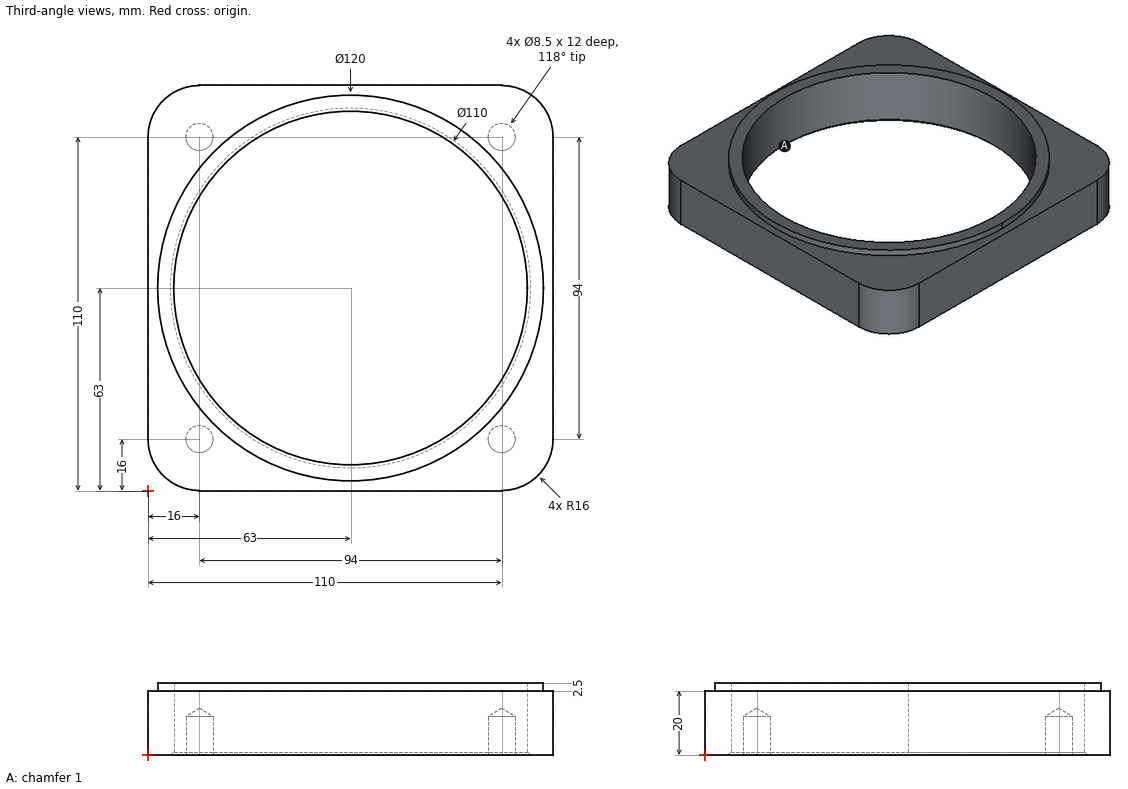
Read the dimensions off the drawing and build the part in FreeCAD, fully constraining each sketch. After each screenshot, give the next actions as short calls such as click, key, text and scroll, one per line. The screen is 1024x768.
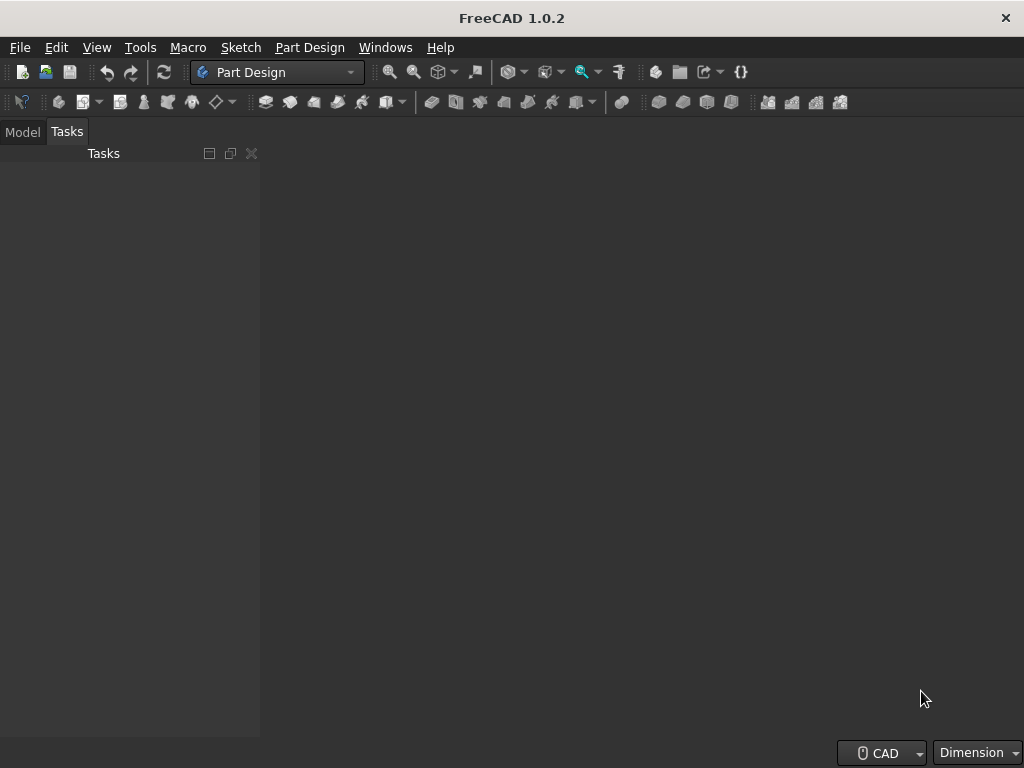
click(22, 72)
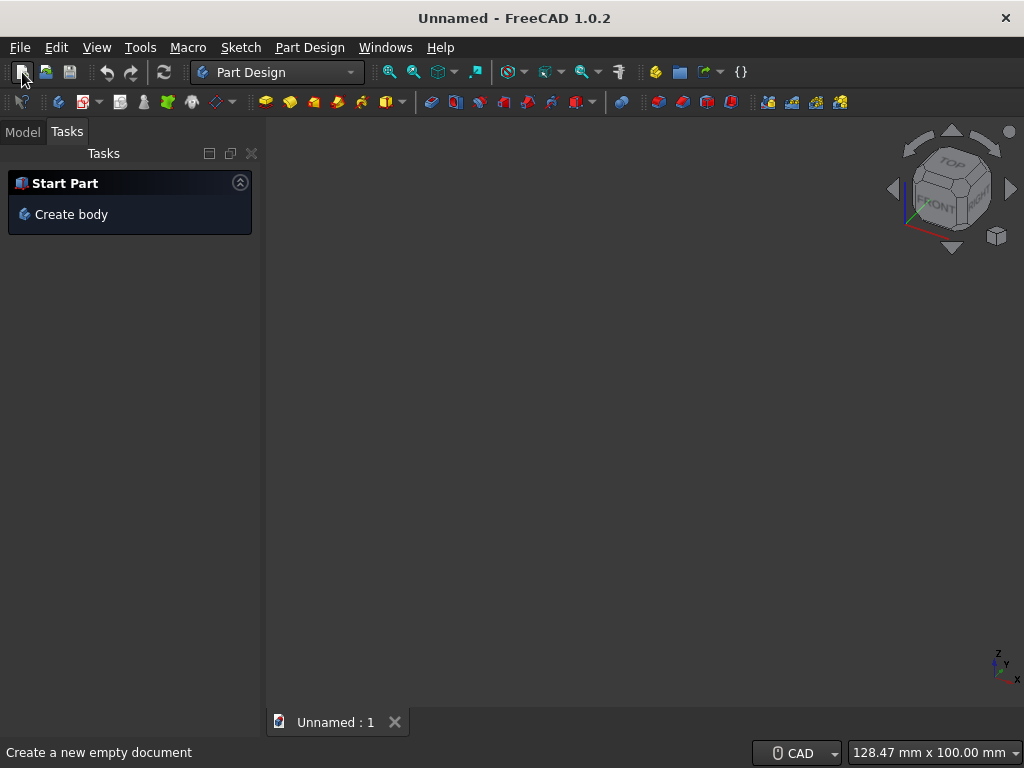
click(84, 102)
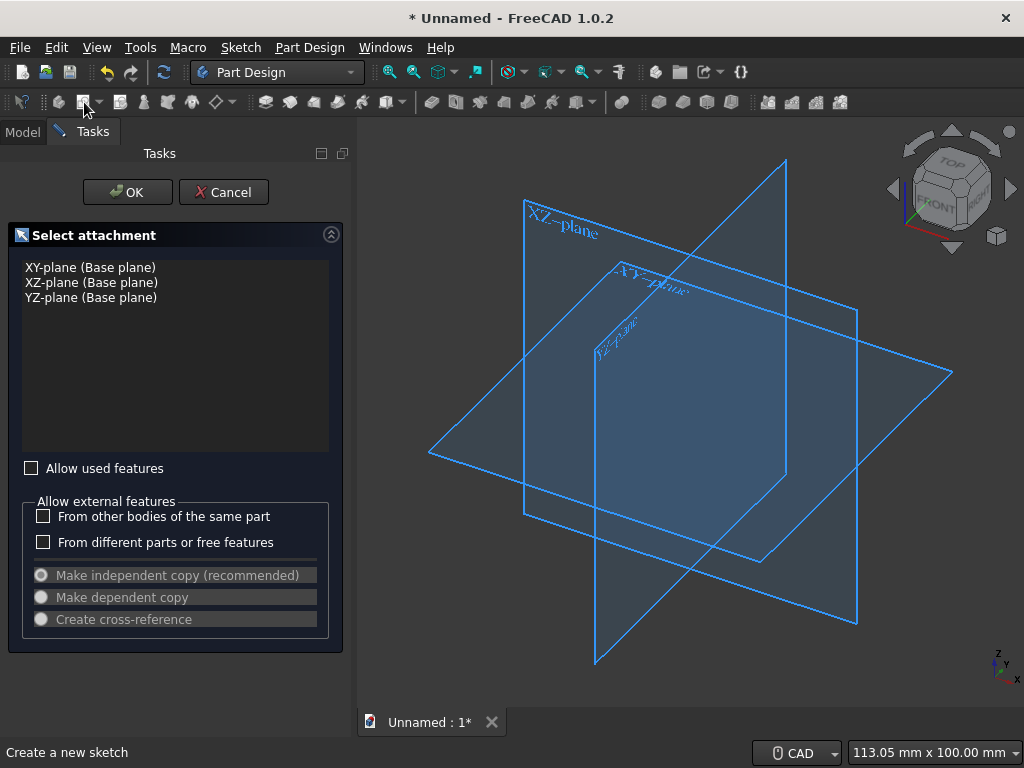
click(82, 268)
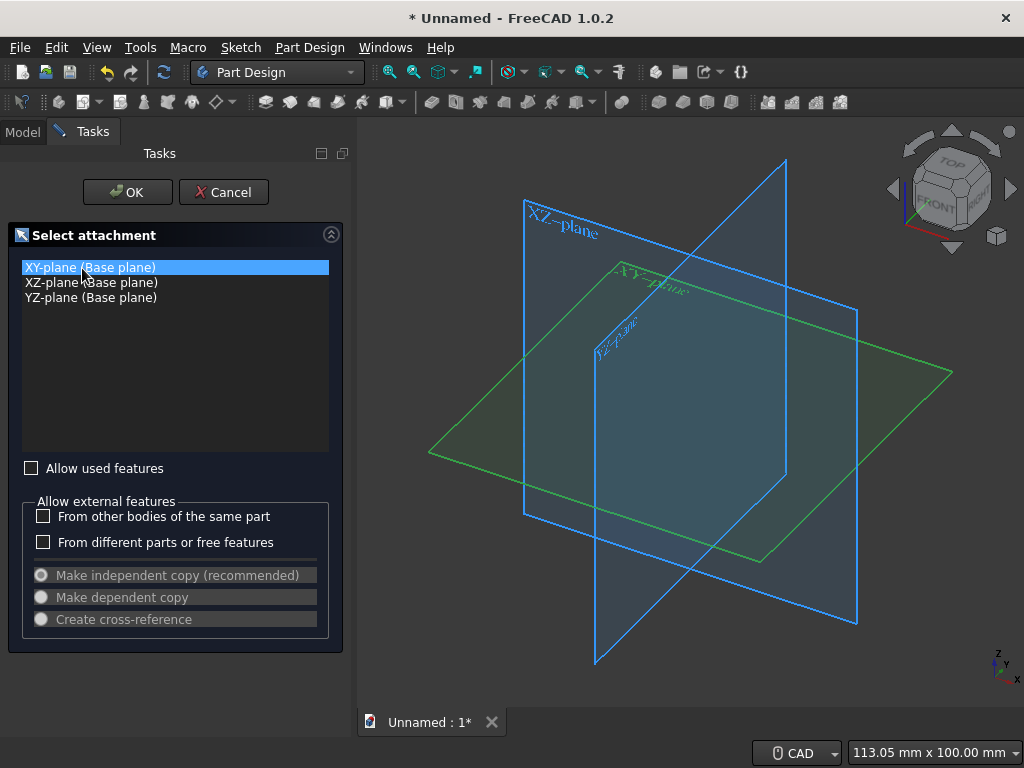
click(128, 192)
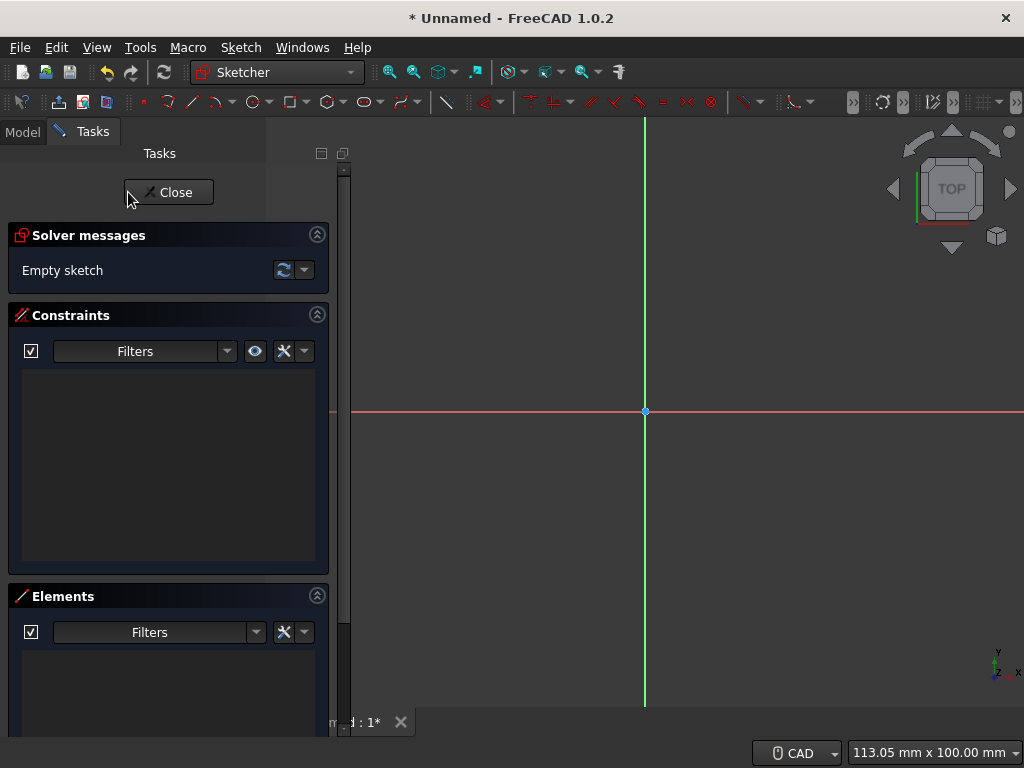
scroll(294, 679, down, 4)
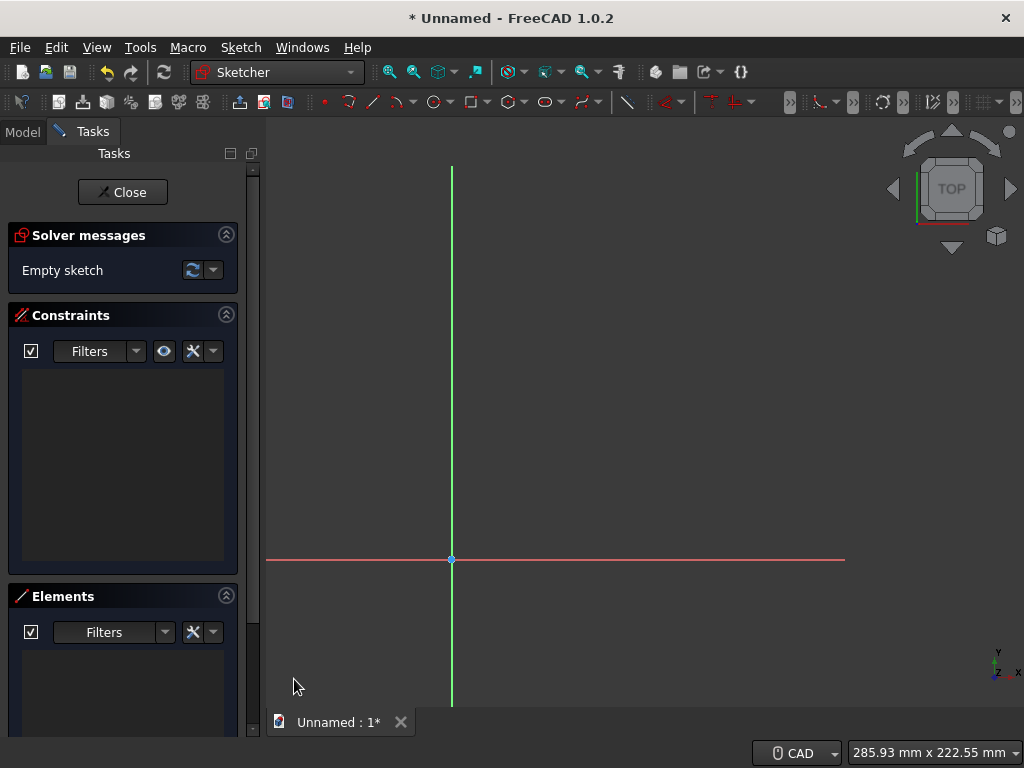
click(374, 102)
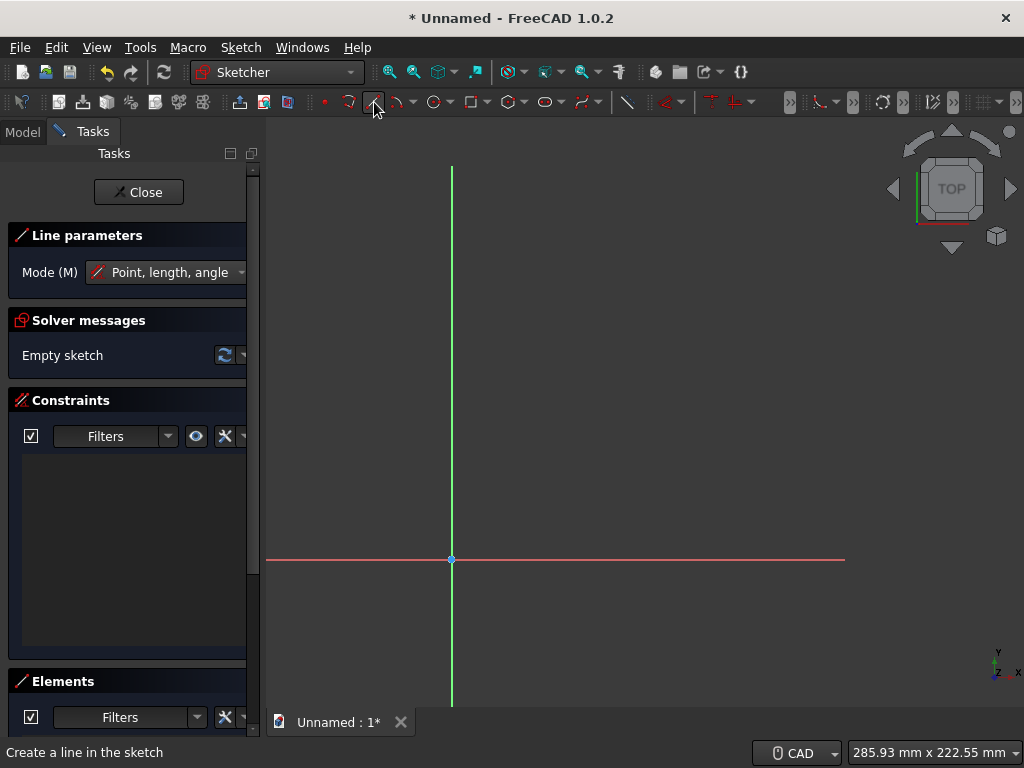
click(494, 560)
click(743, 551)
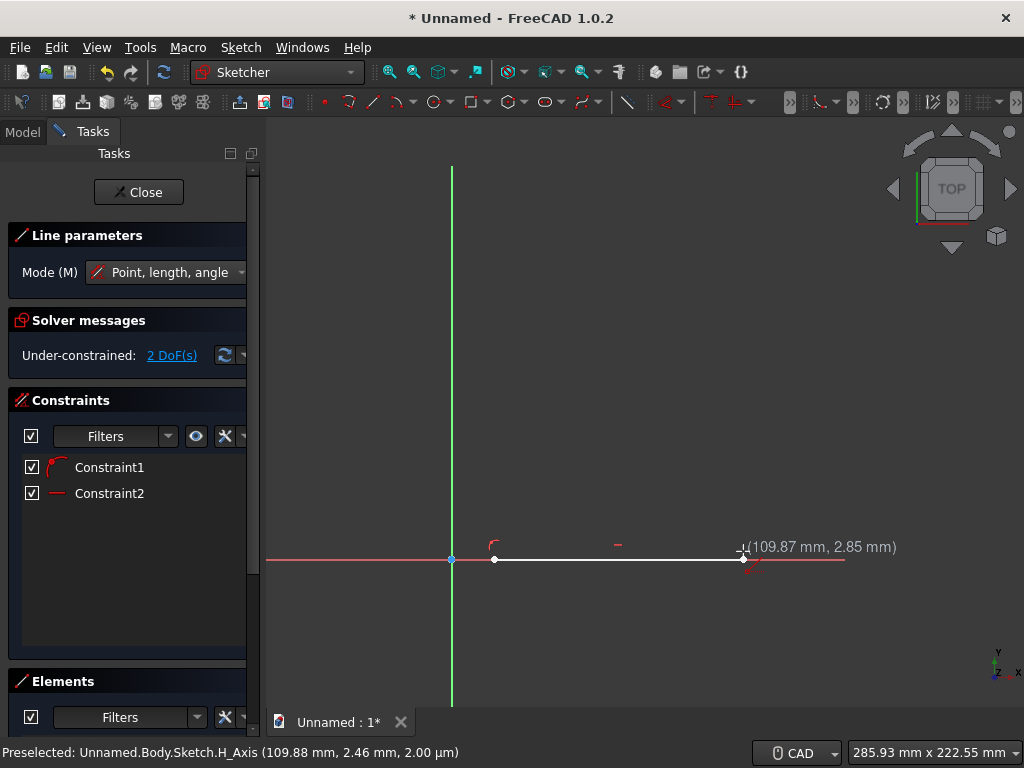
click(786, 517)
click(786, 268)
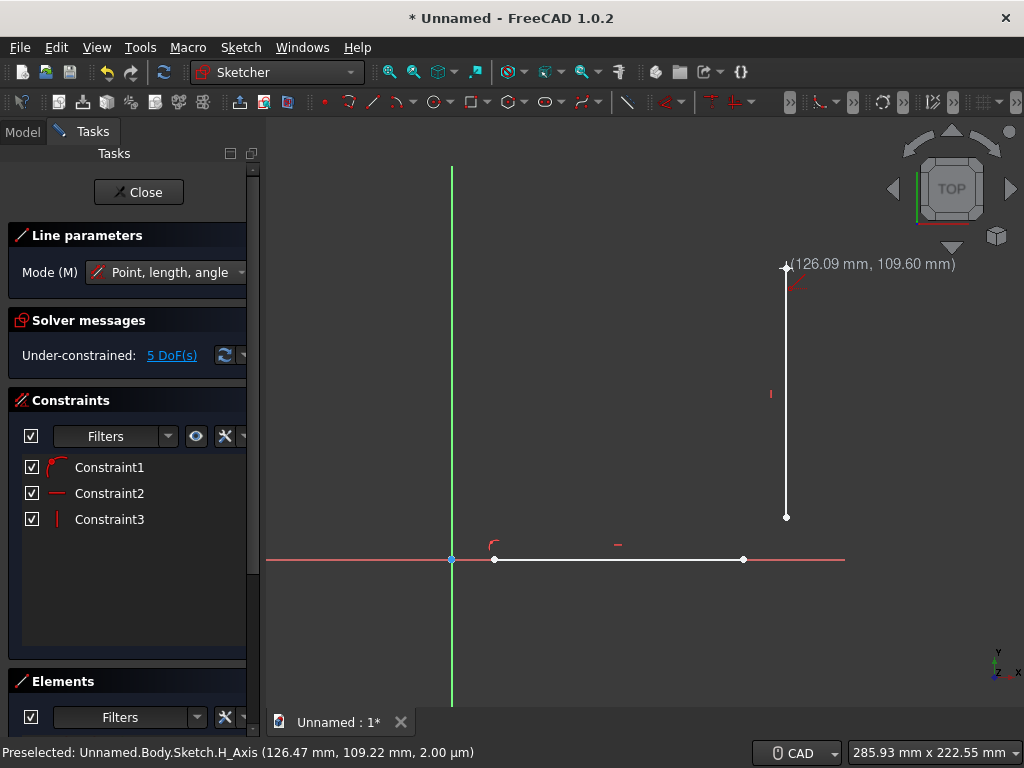
click(743, 226)
click(494, 226)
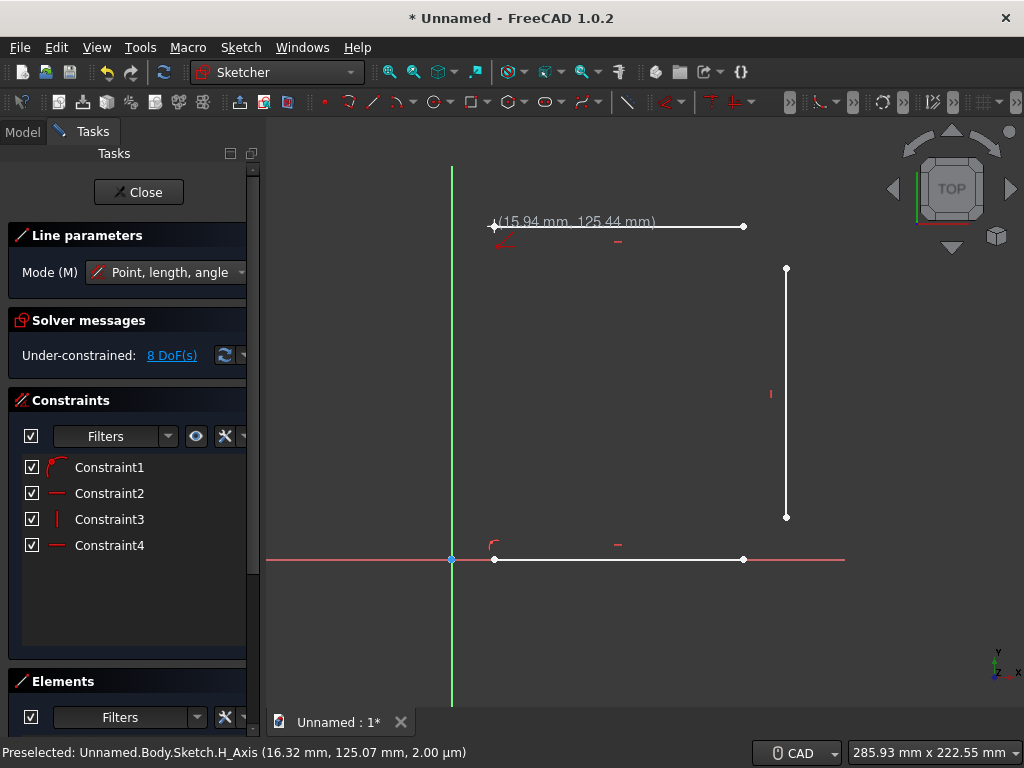
click(452, 268)
click(461, 517)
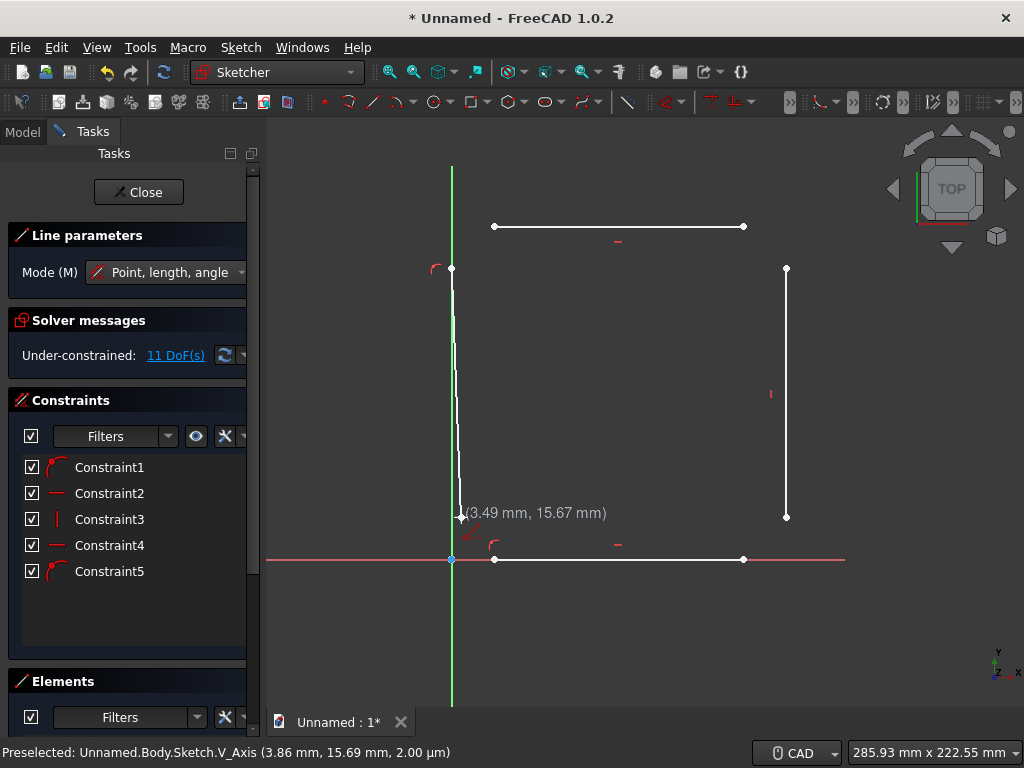
key(g)
key(3)
key(a)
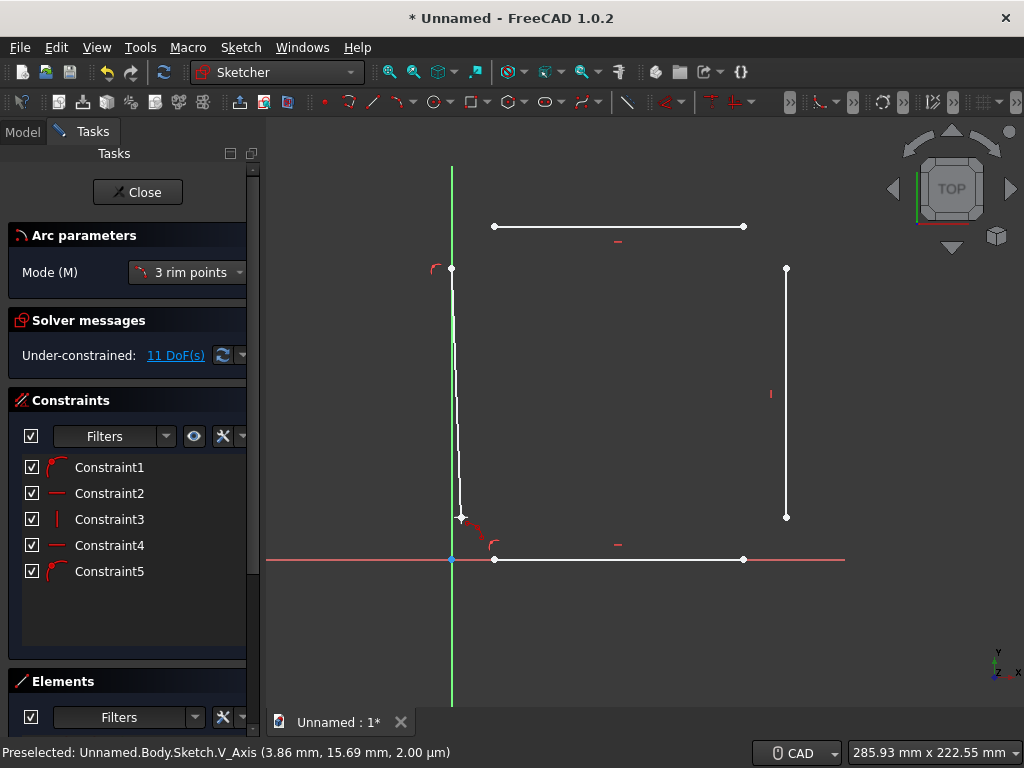
click(743, 560)
click(786, 518)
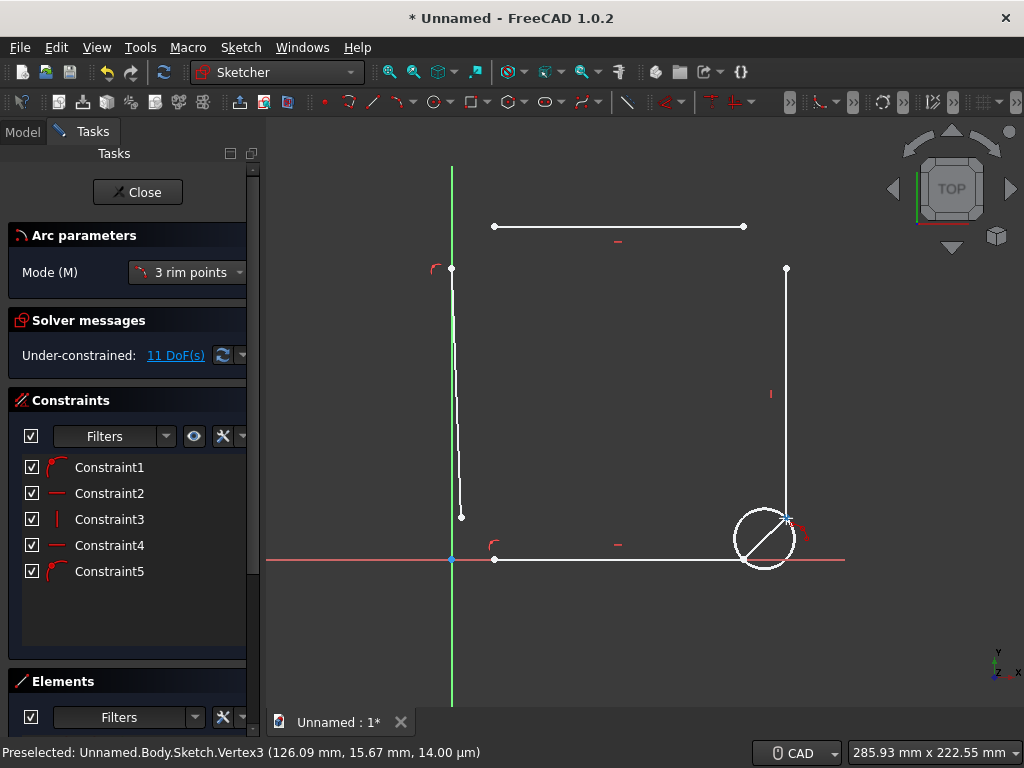
scroll(773, 547, up, 2)